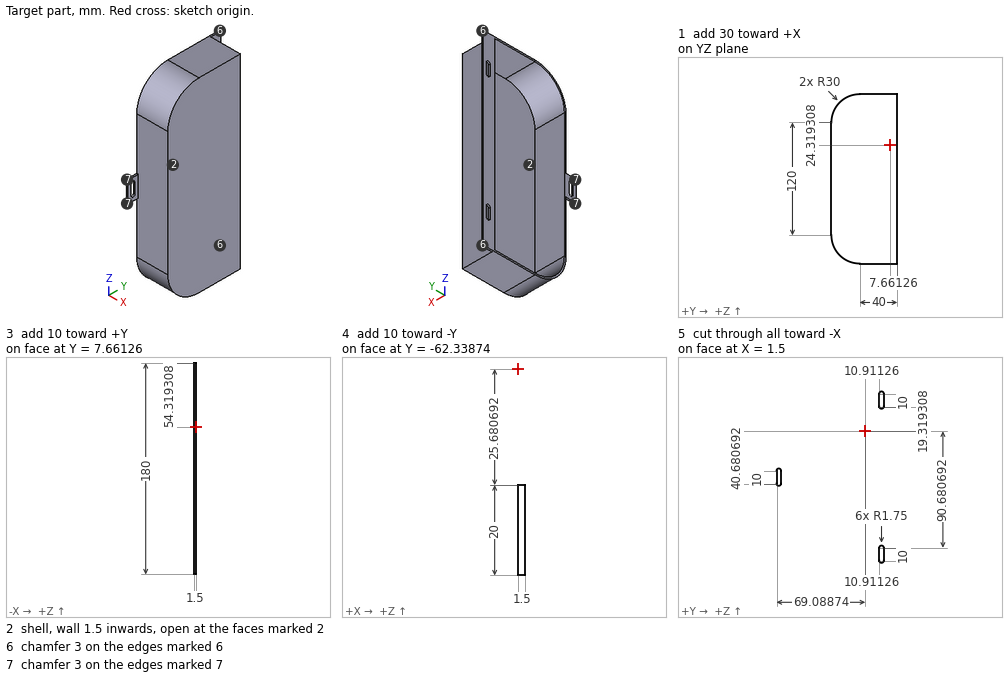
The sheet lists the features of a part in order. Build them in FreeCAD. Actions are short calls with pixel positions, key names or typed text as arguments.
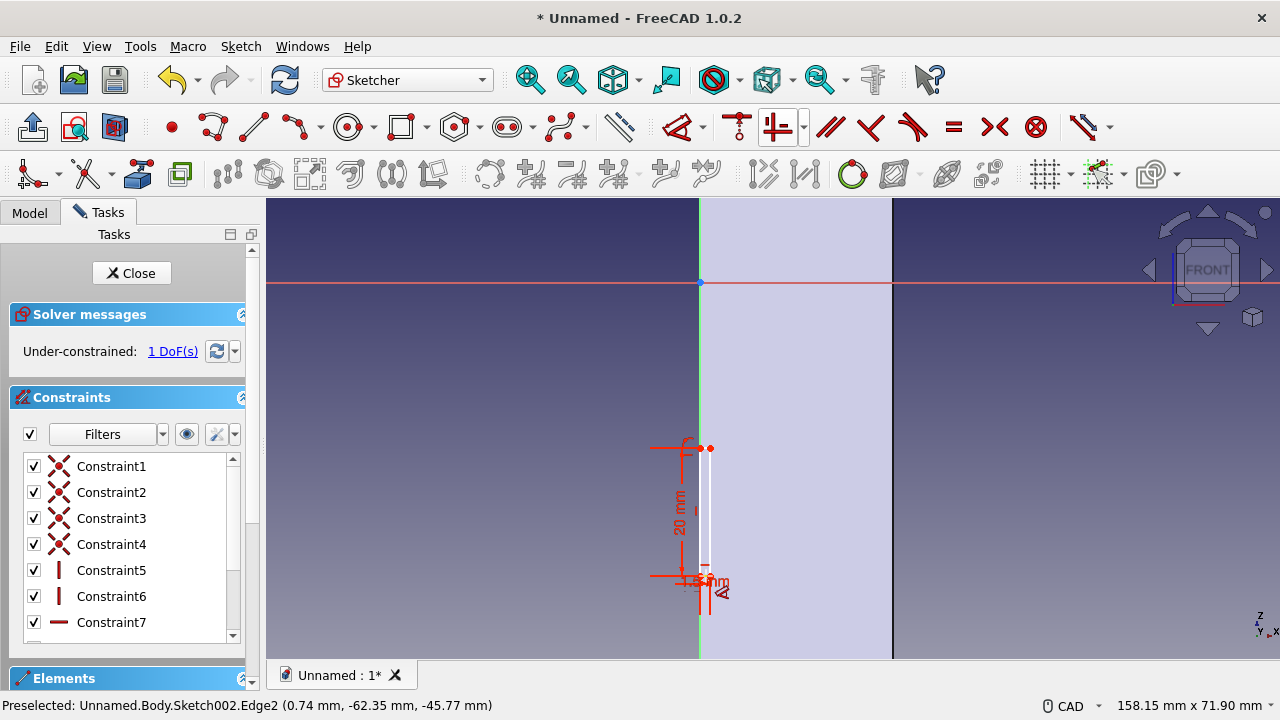
scroll(700, 448, up, 2)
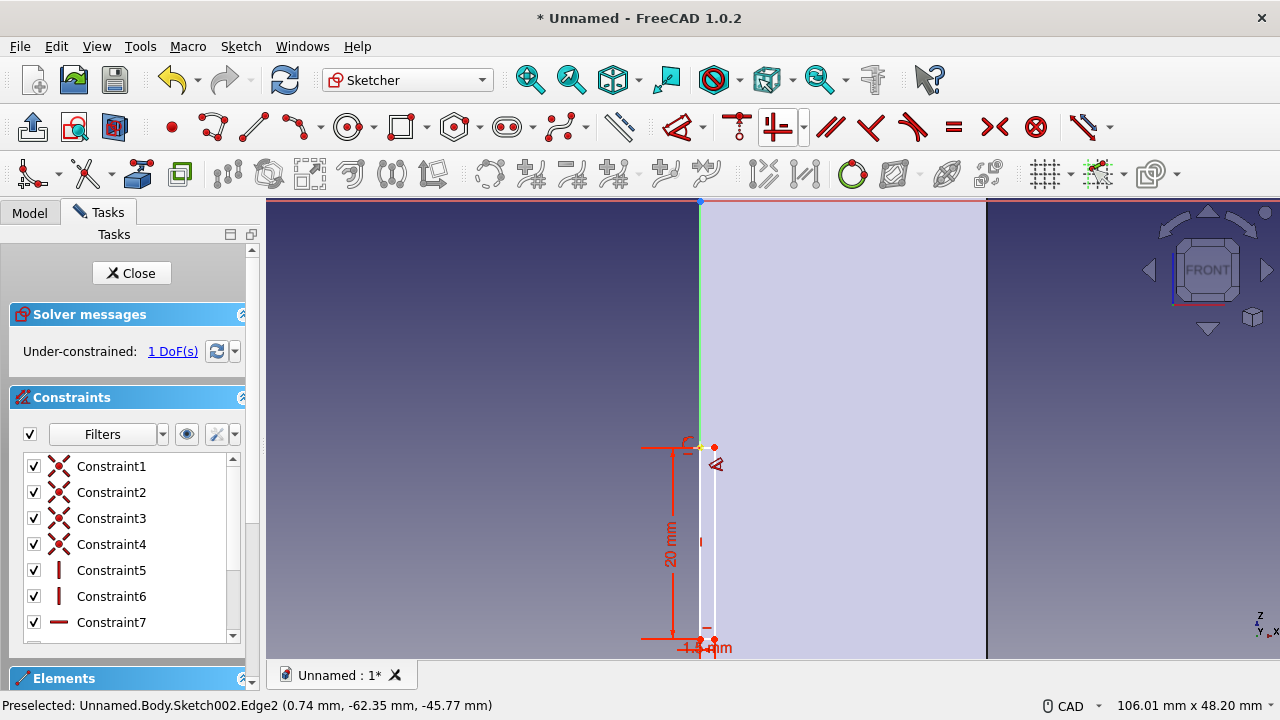
click(700, 448)
click(666, 337)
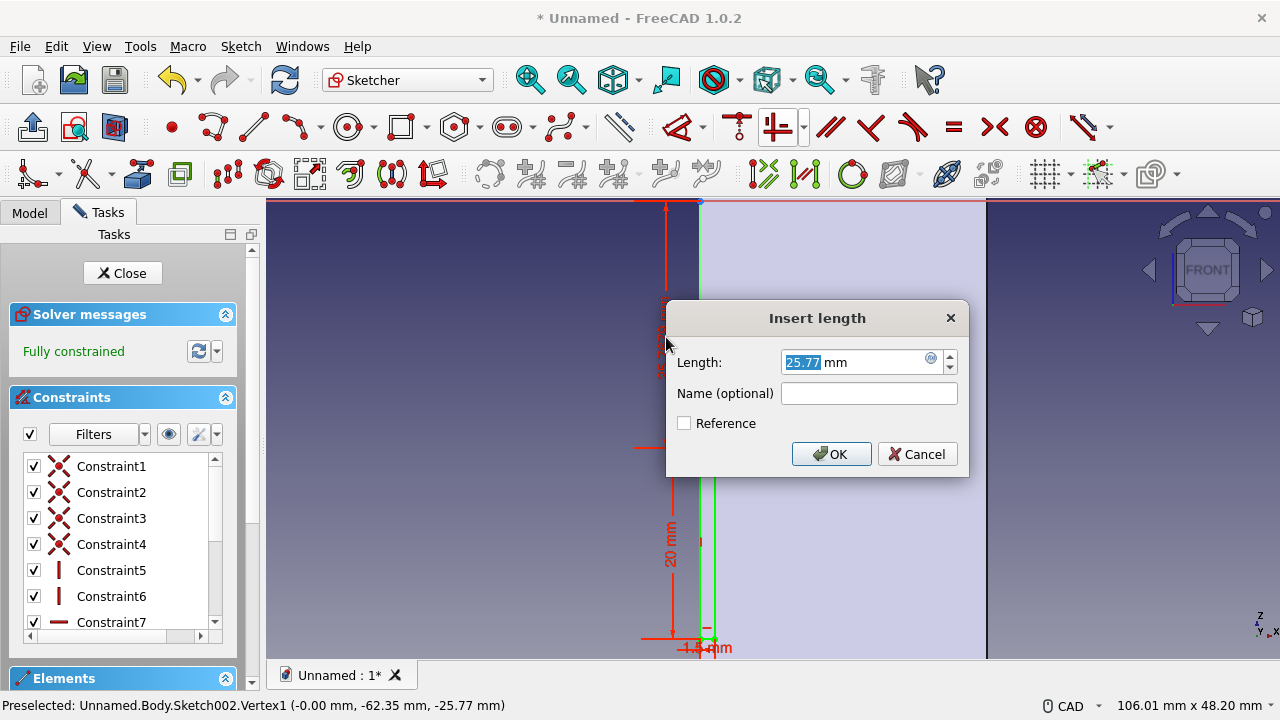
text(25.680692)
key(Return)
key(Escape)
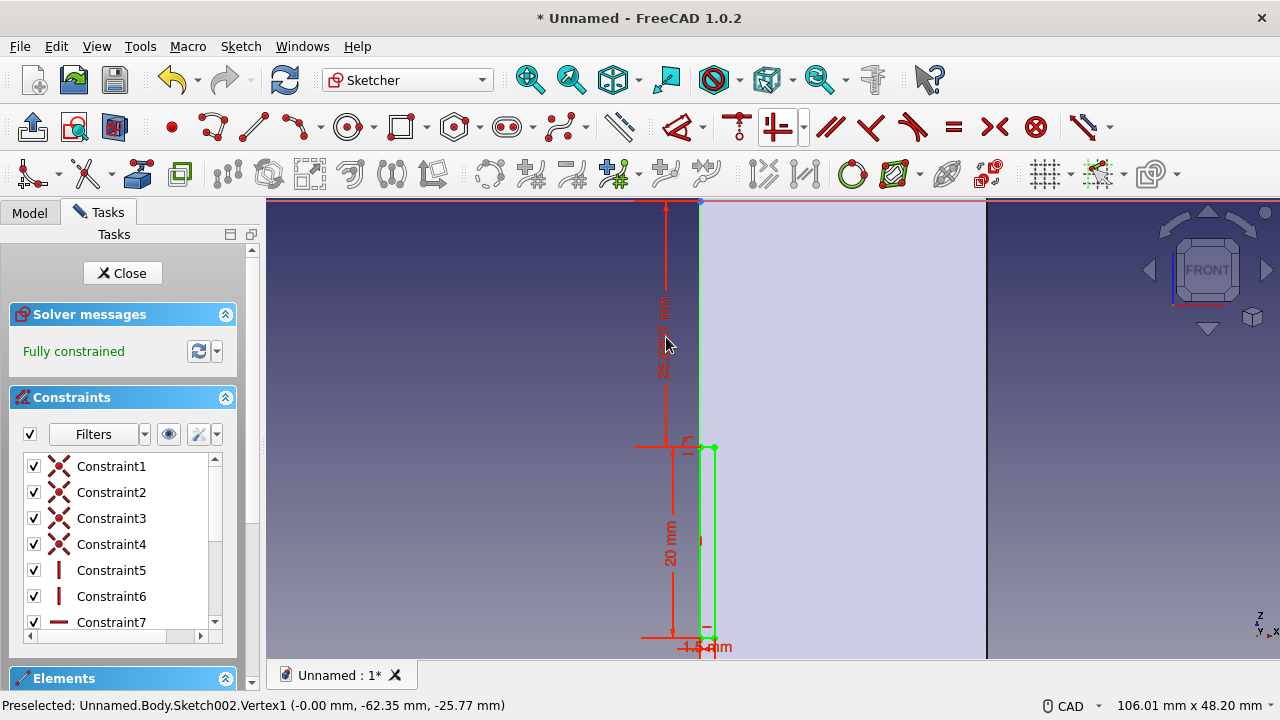
click(123, 273)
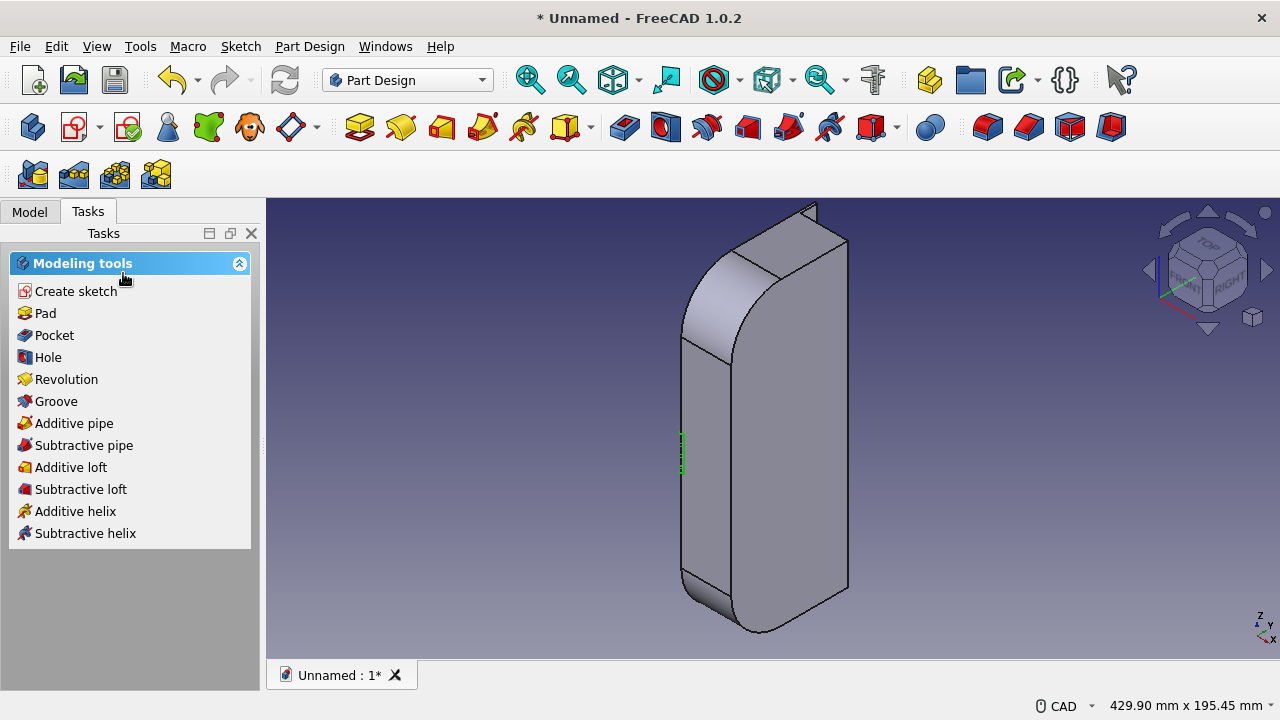
click(360, 128)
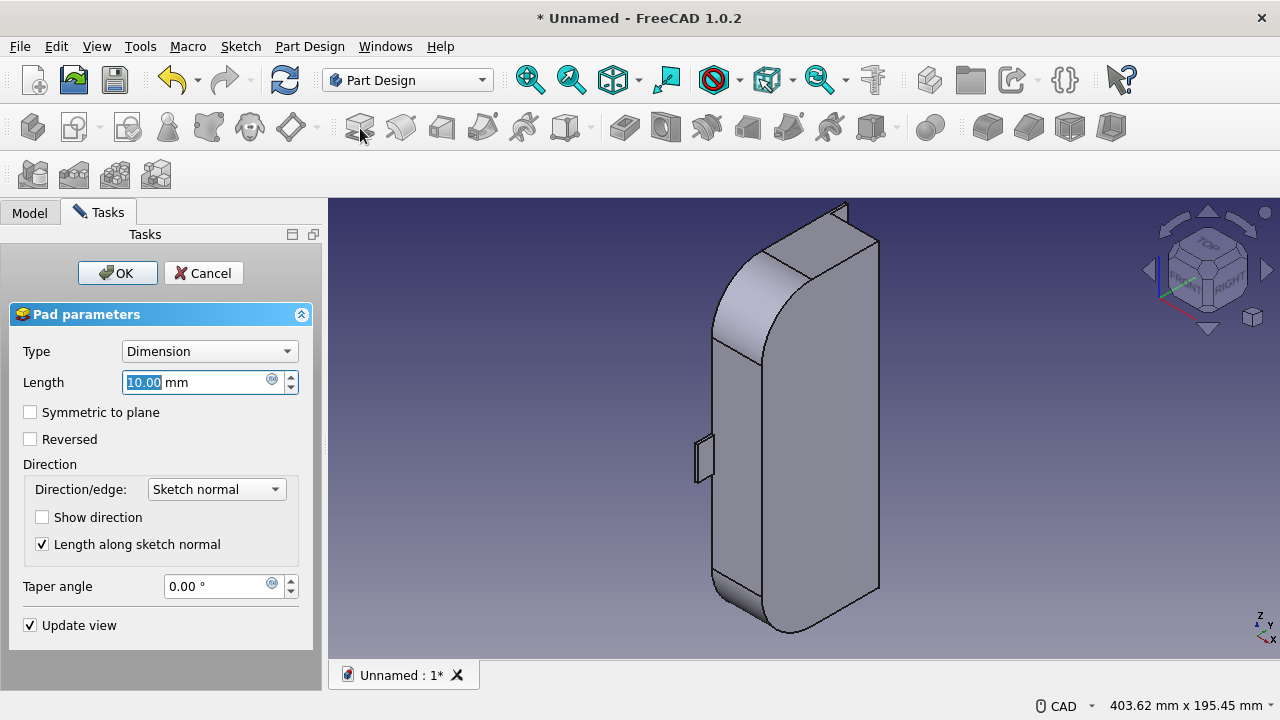
text(10)
key(Tab)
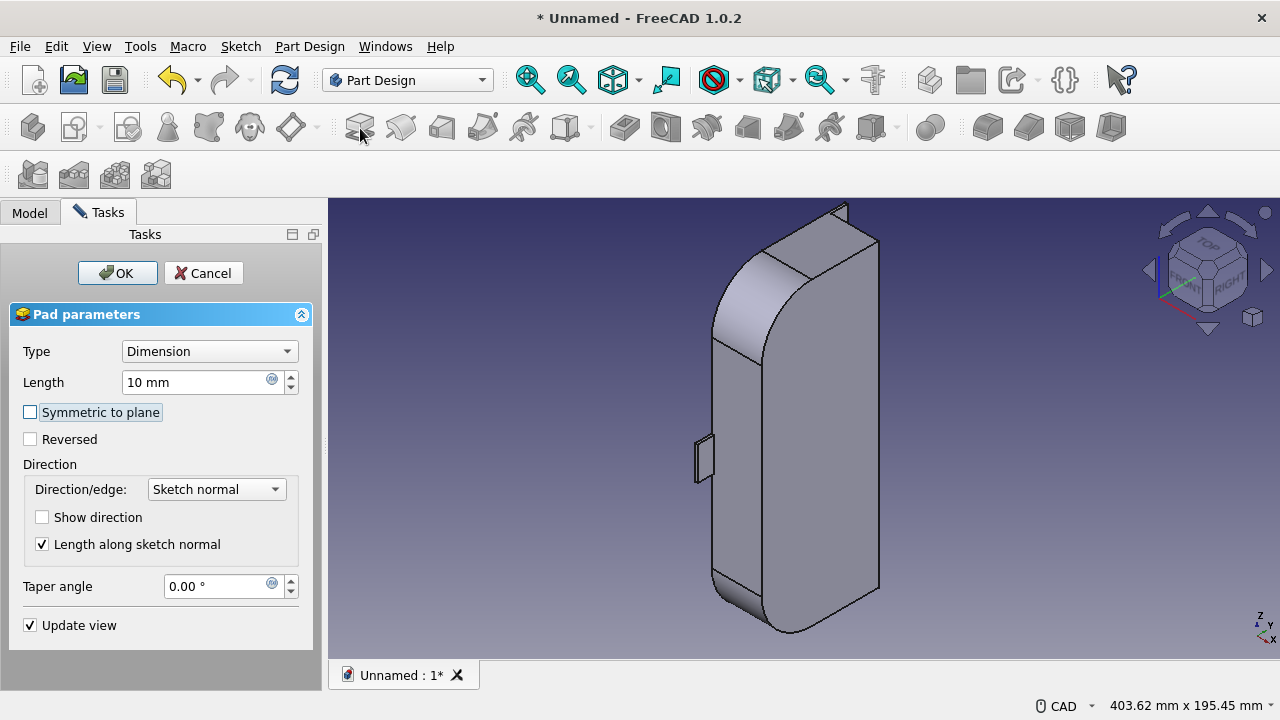
click(118, 273)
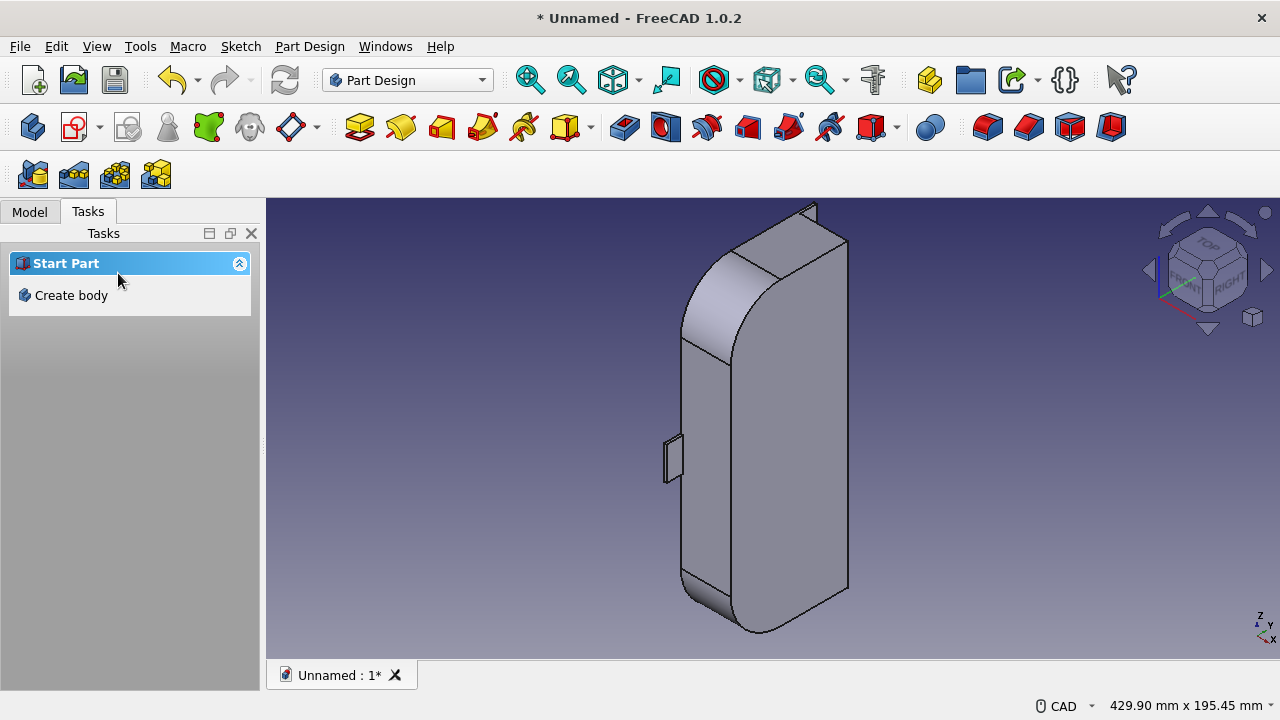
click(531, 80)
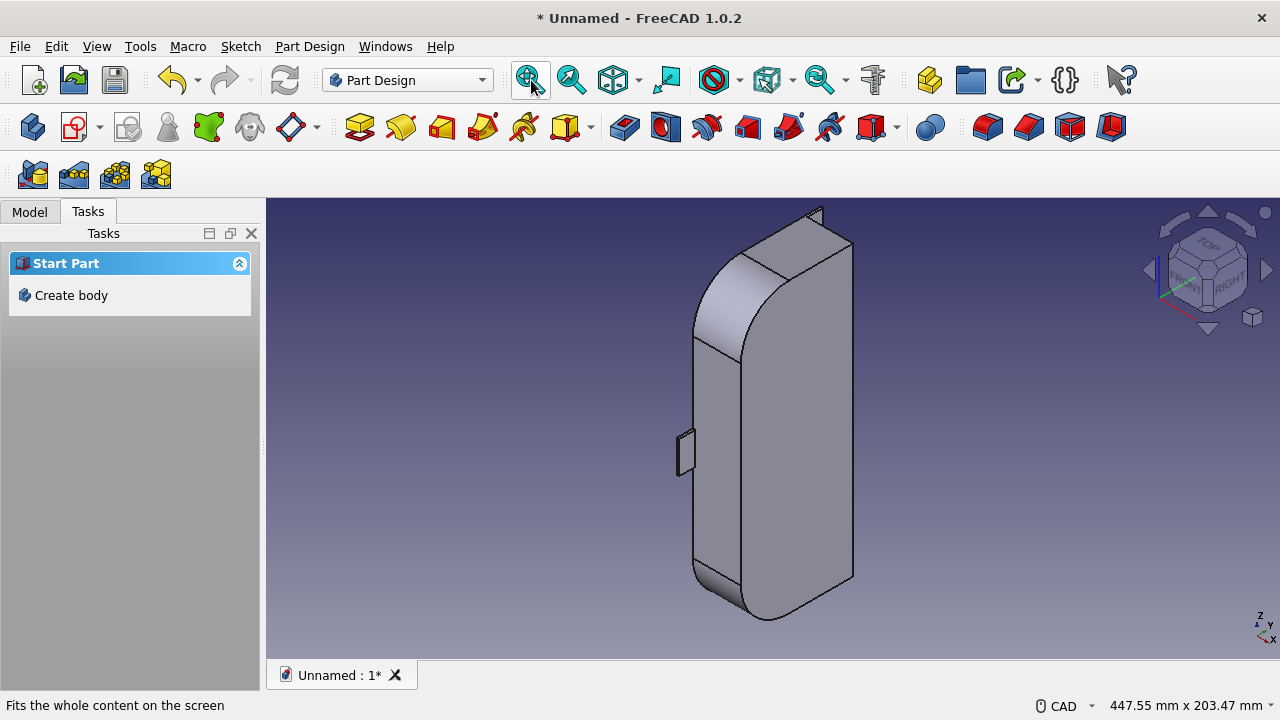
key(3)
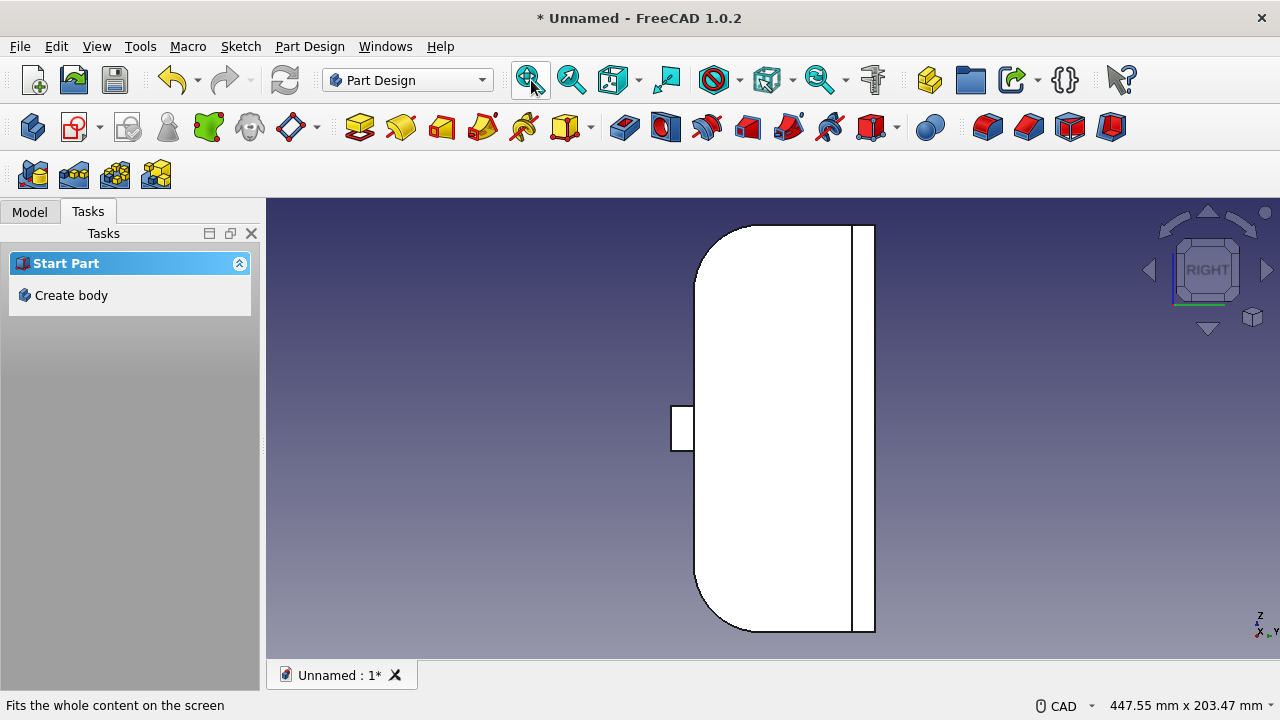
click(864, 311)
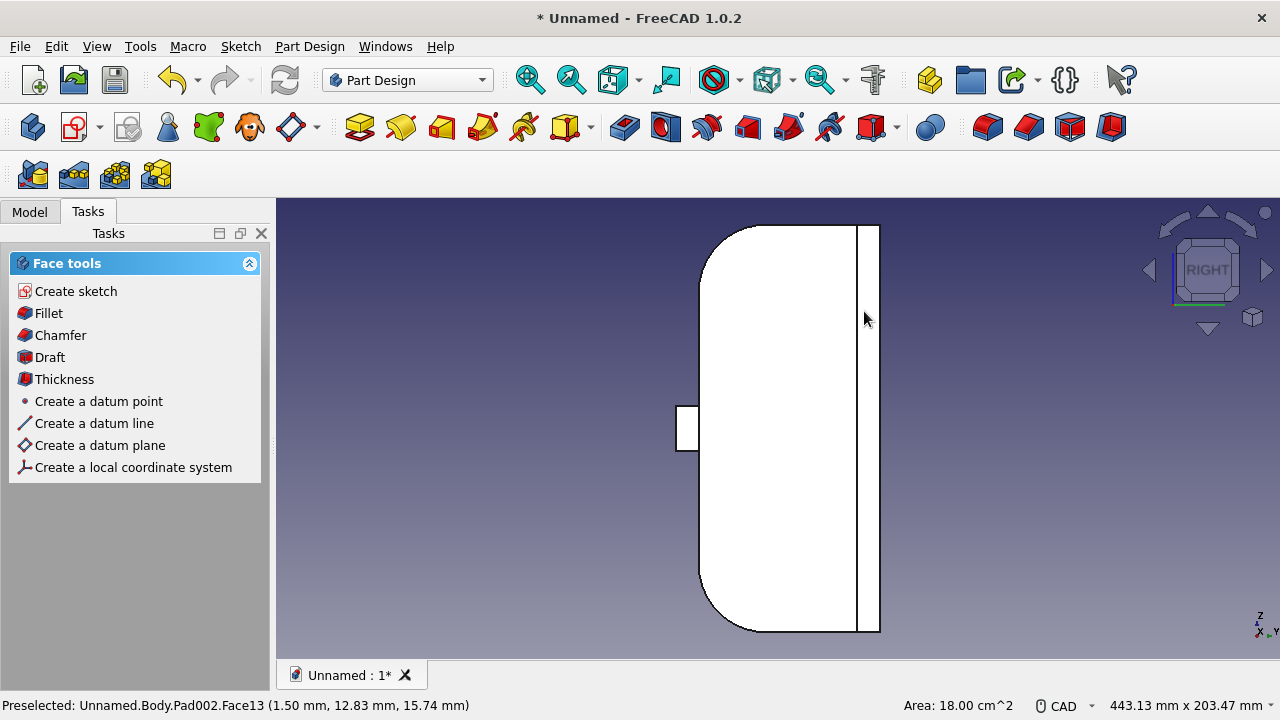
click(74, 128)